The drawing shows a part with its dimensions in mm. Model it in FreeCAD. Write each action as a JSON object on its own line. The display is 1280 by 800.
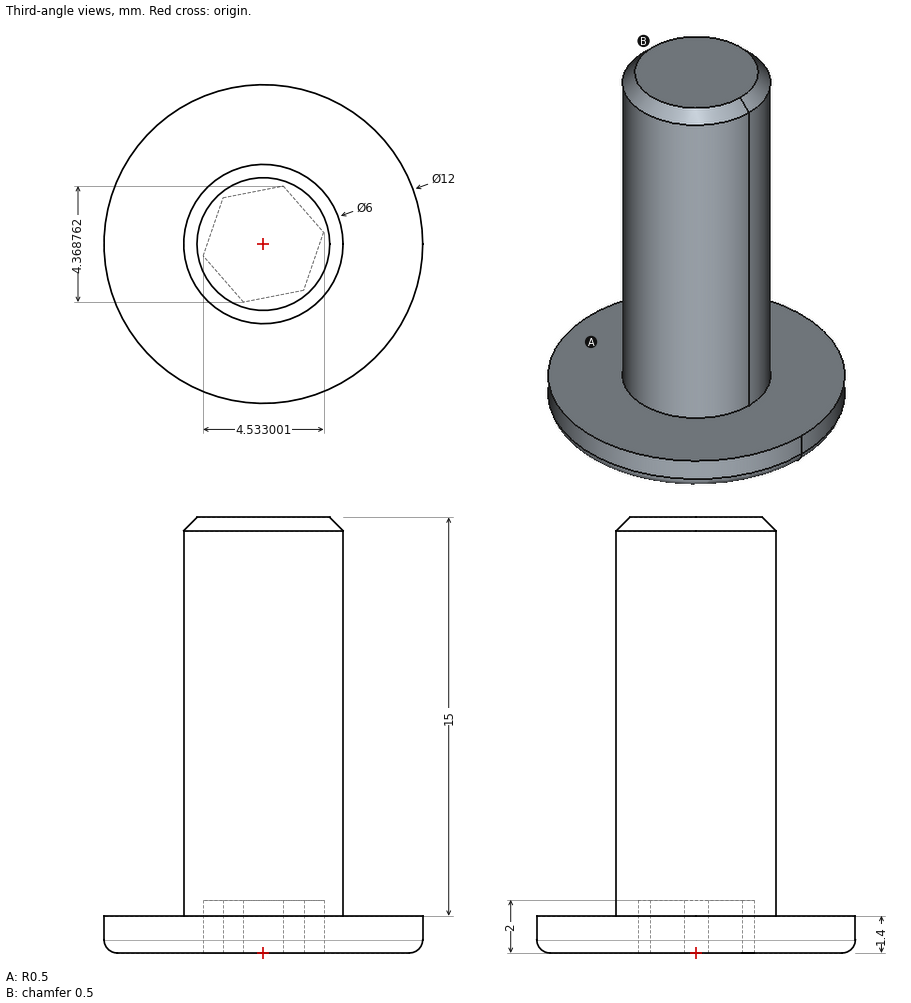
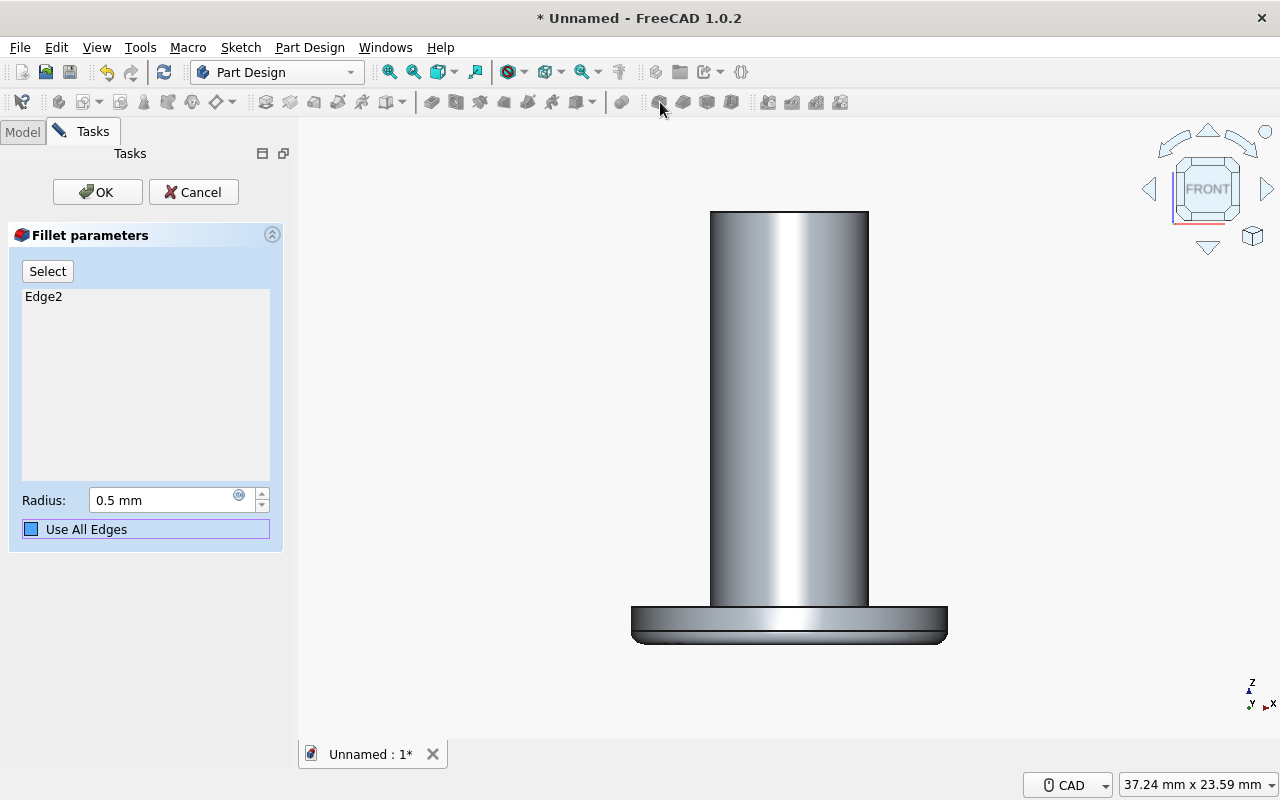
{"action": "left_click", "coordinate": [98, 192]}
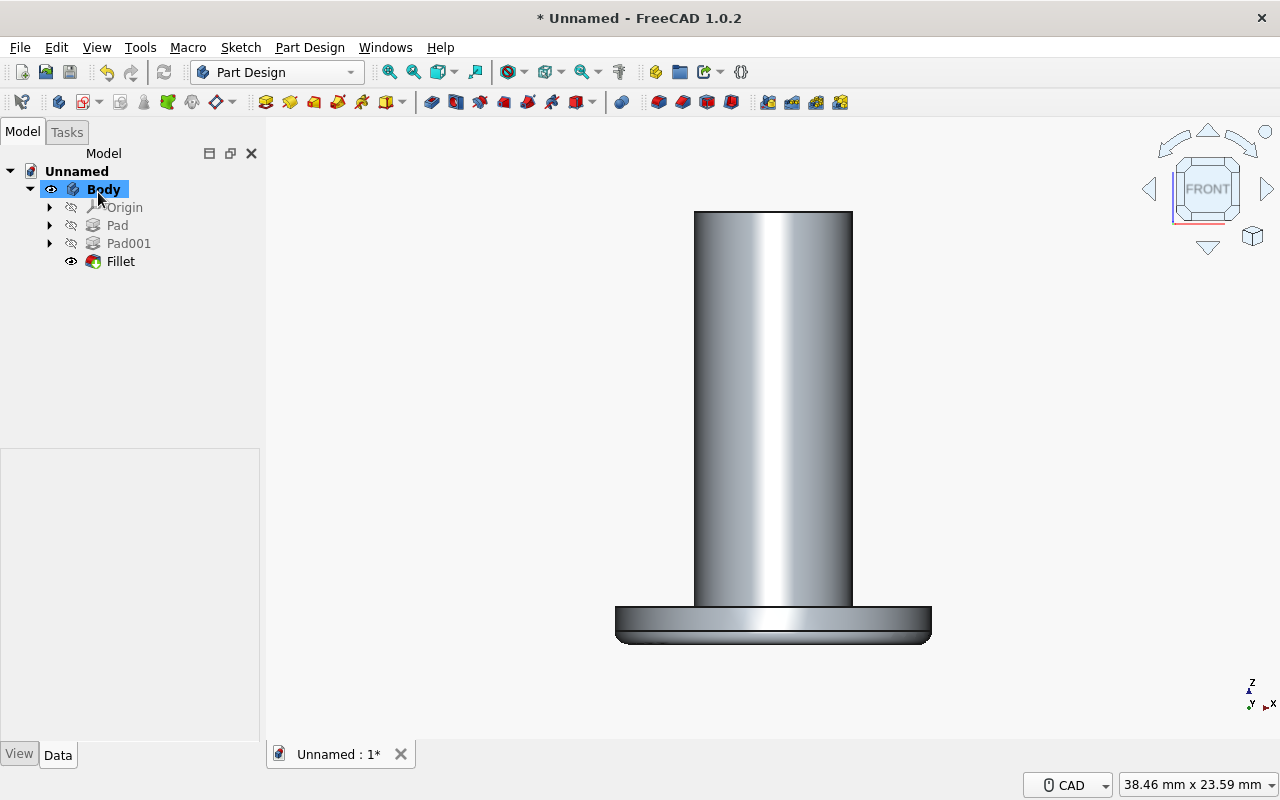
{"action": "left_click", "coordinate": [84, 102]}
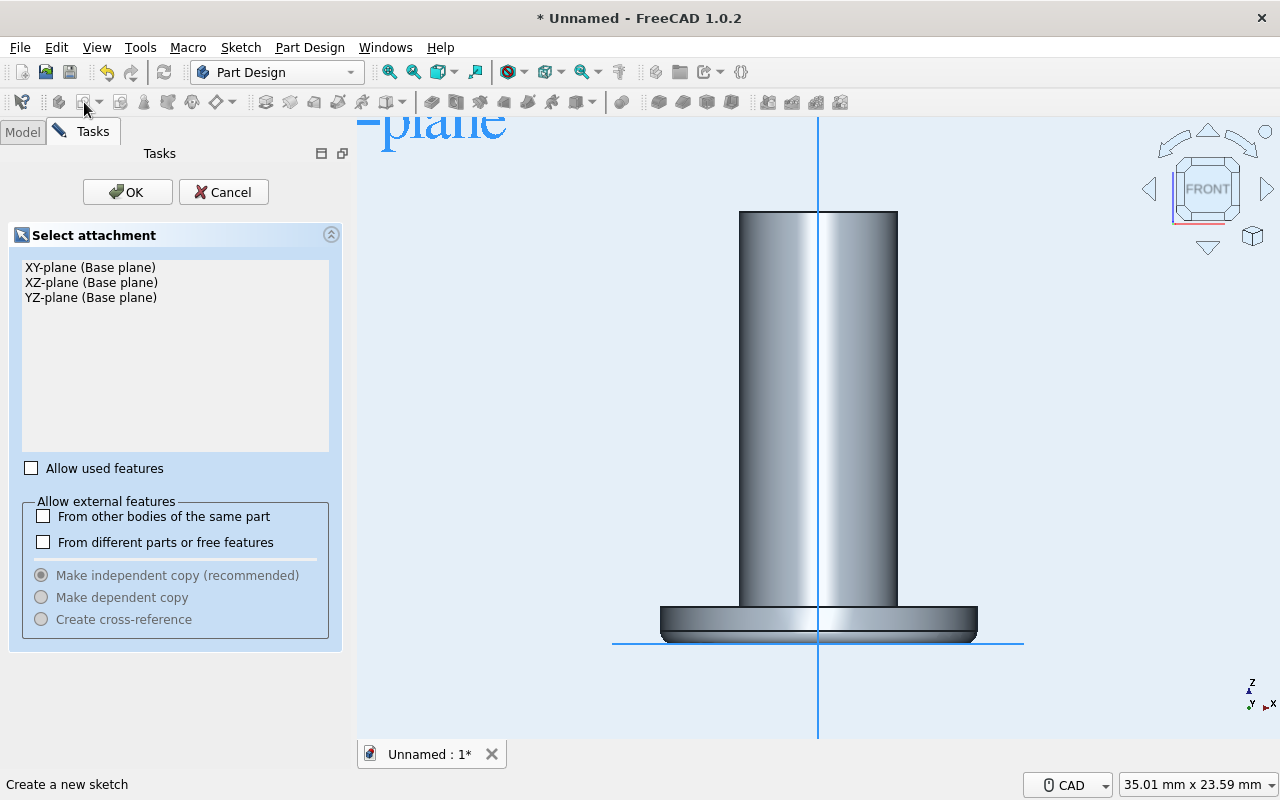
{"action": "left_click", "coordinate": [82, 268]}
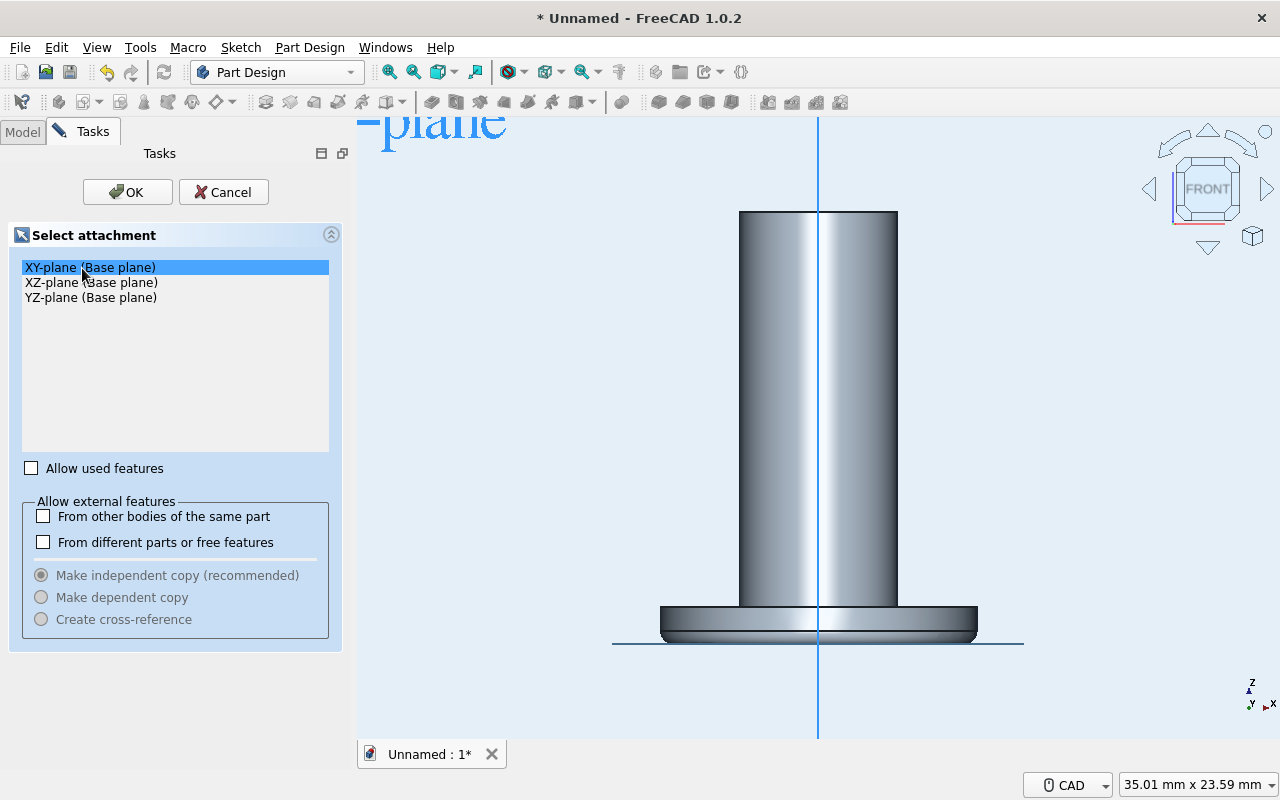
{"action": "left_click", "coordinate": [128, 192]}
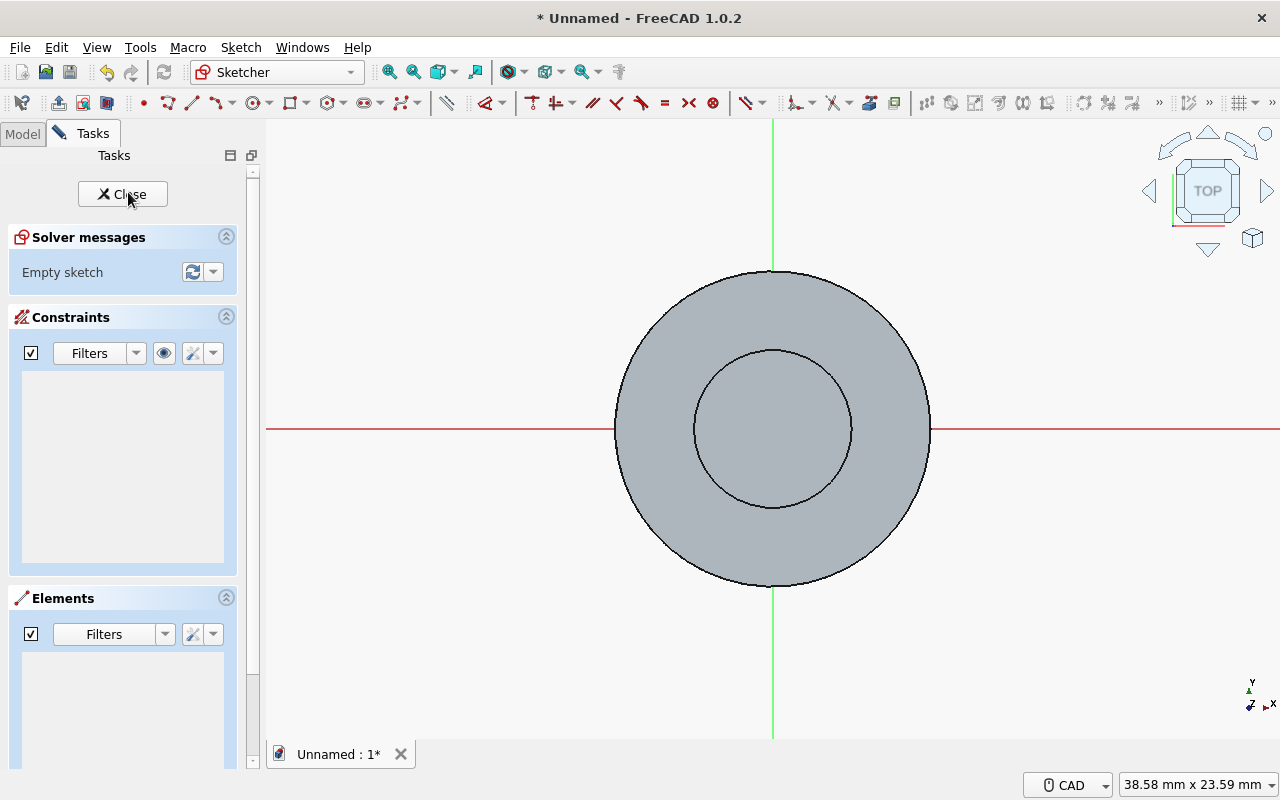
{"action": "left_click", "coordinate": [108, 104]}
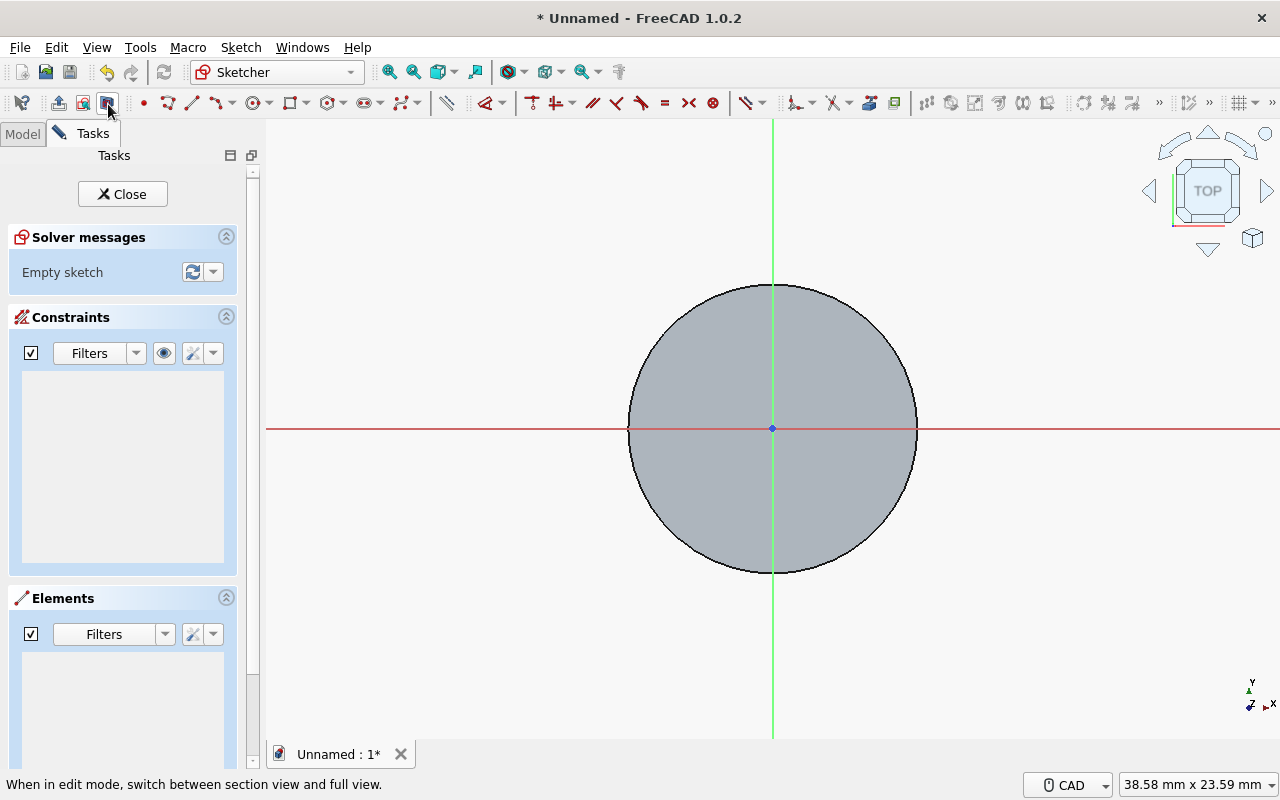
{"action": "scroll", "coordinate": [802, 429], "scroll_direction": "up", "scroll_amount": 6}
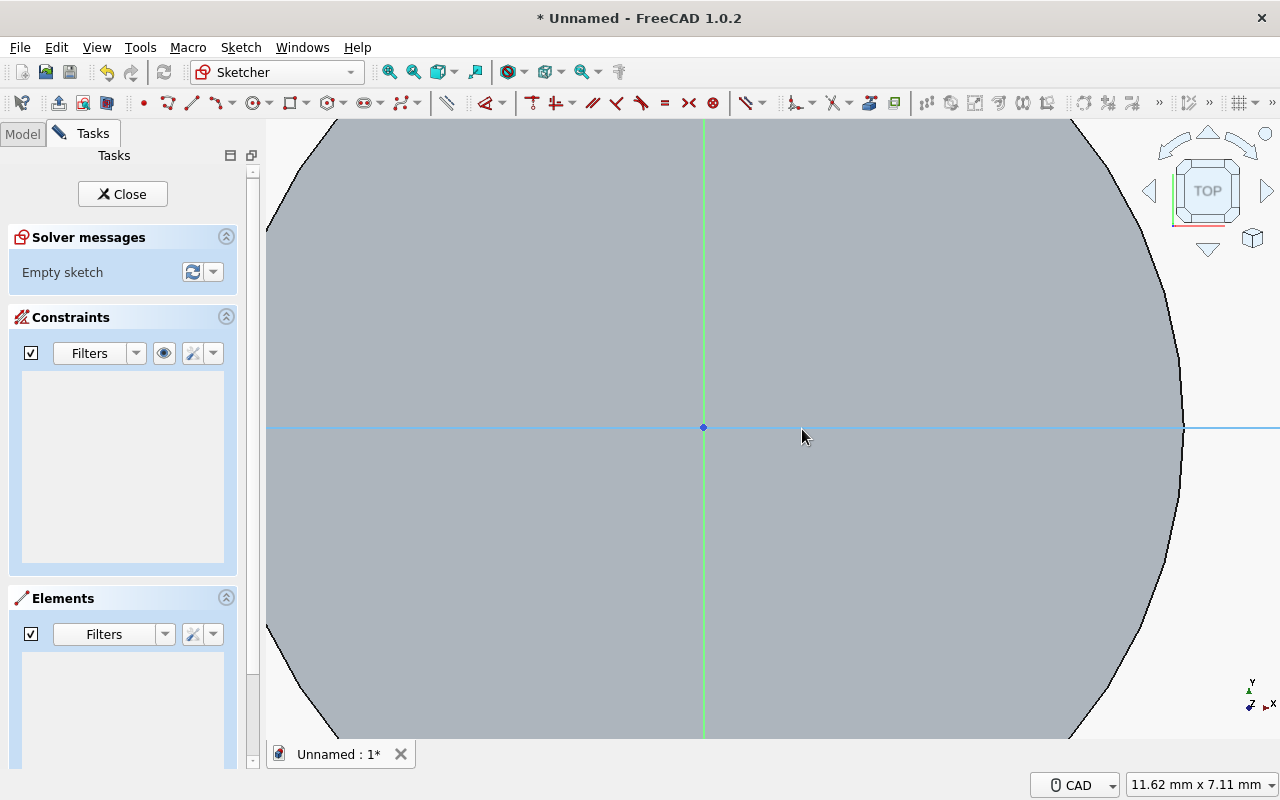
{"action": "left_click", "coordinate": [328, 104]}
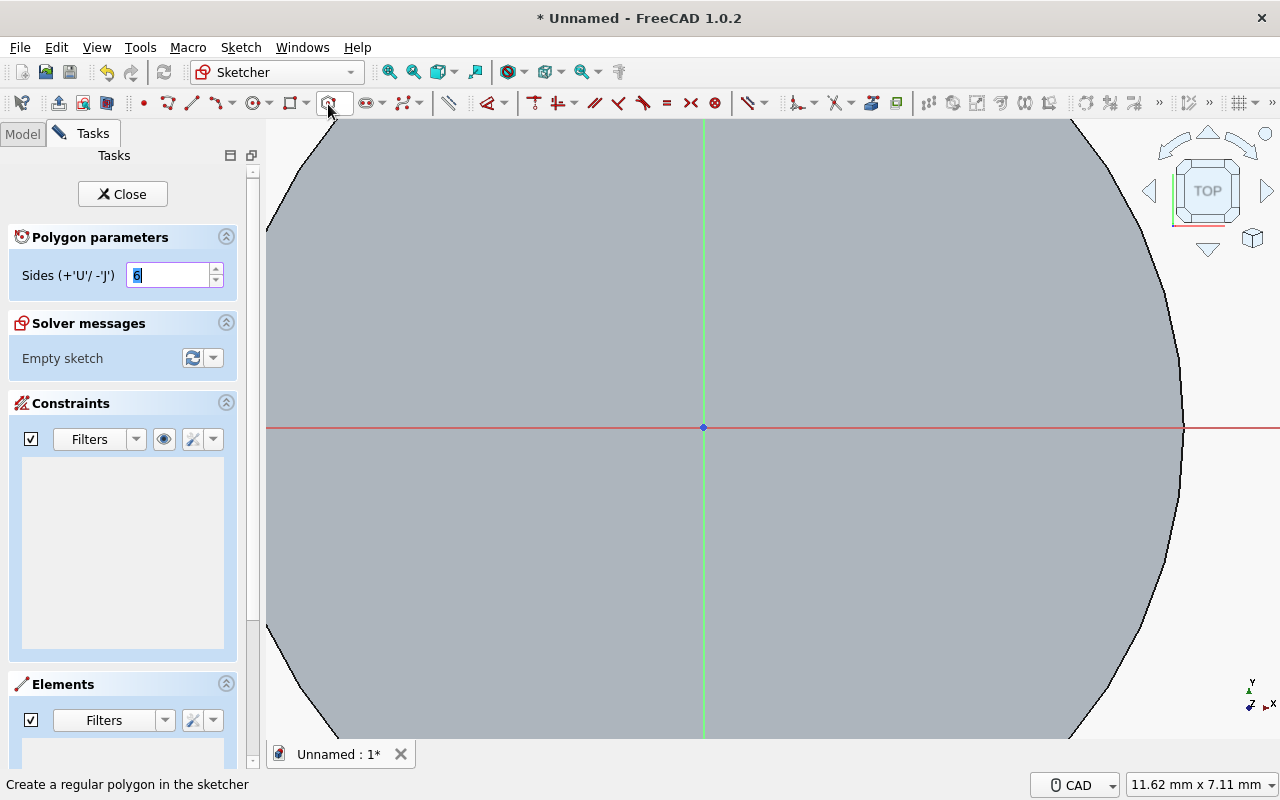
{"action": "left_click", "coordinate": [704, 428]}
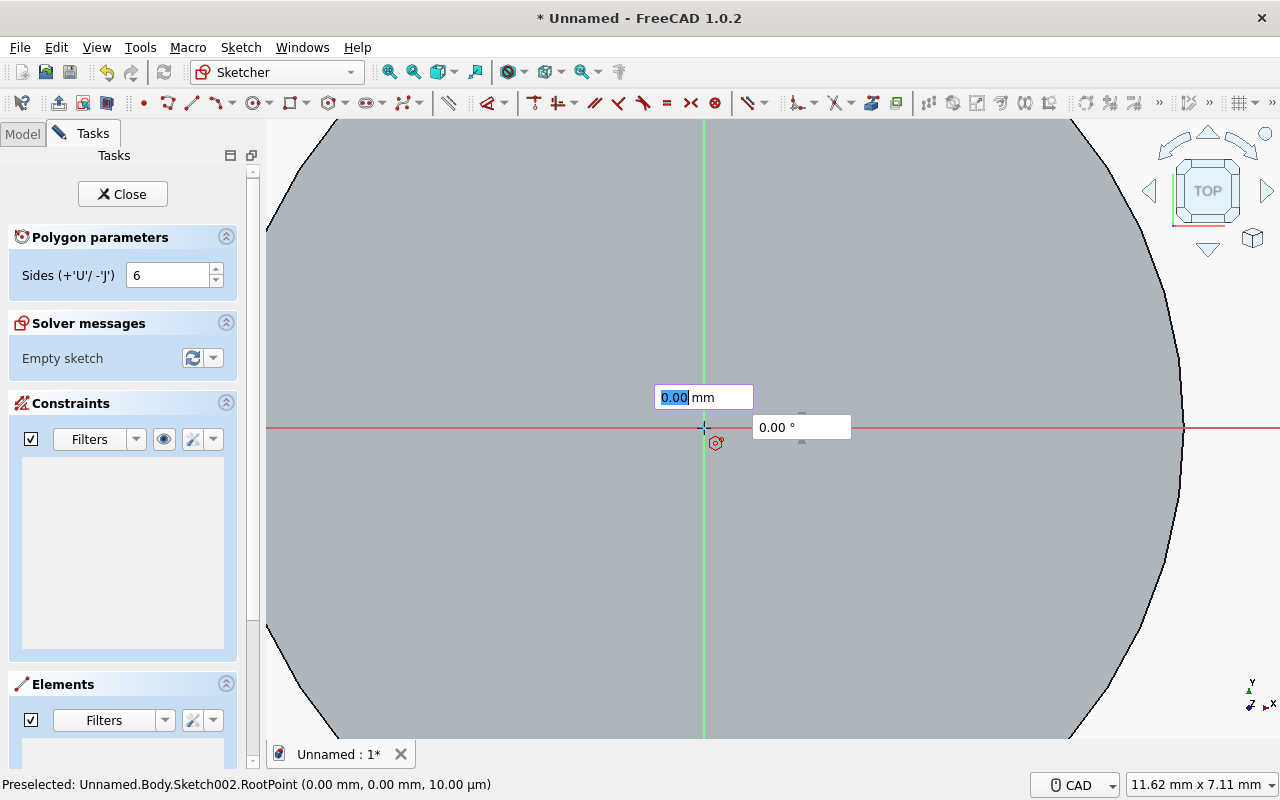
{"action": "left_click", "coordinate": [572, 276]}
{"action": "right_click", "coordinate": [572, 276]}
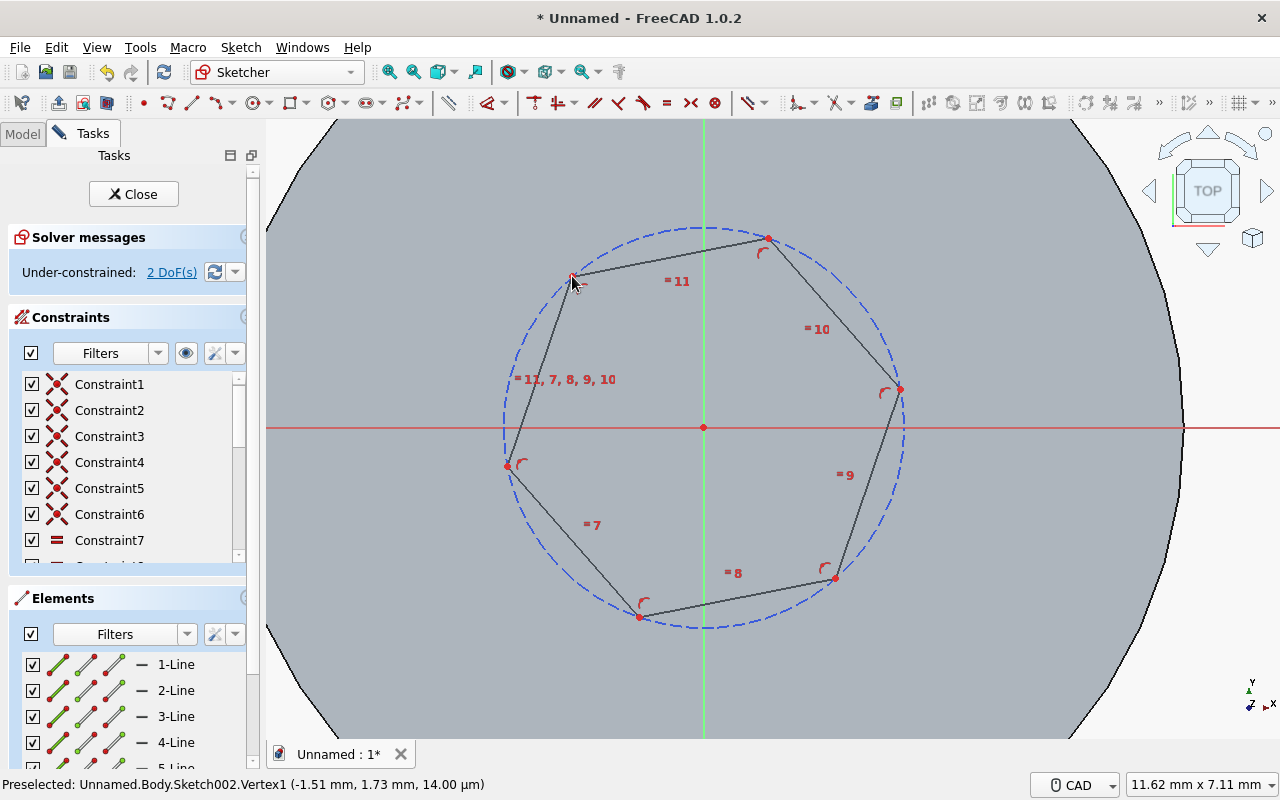
{"action": "left_click", "coordinate": [507, 467]}